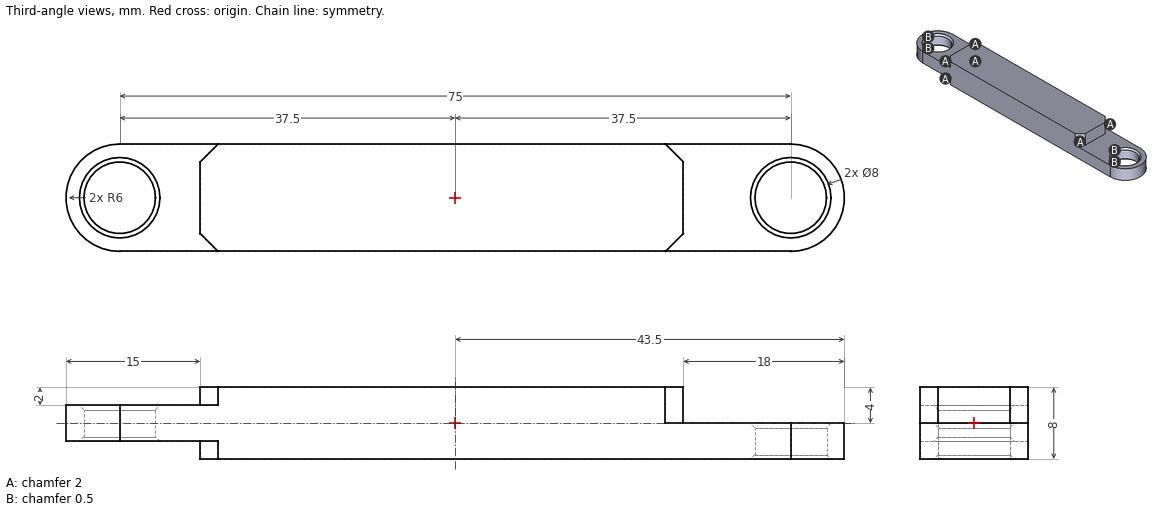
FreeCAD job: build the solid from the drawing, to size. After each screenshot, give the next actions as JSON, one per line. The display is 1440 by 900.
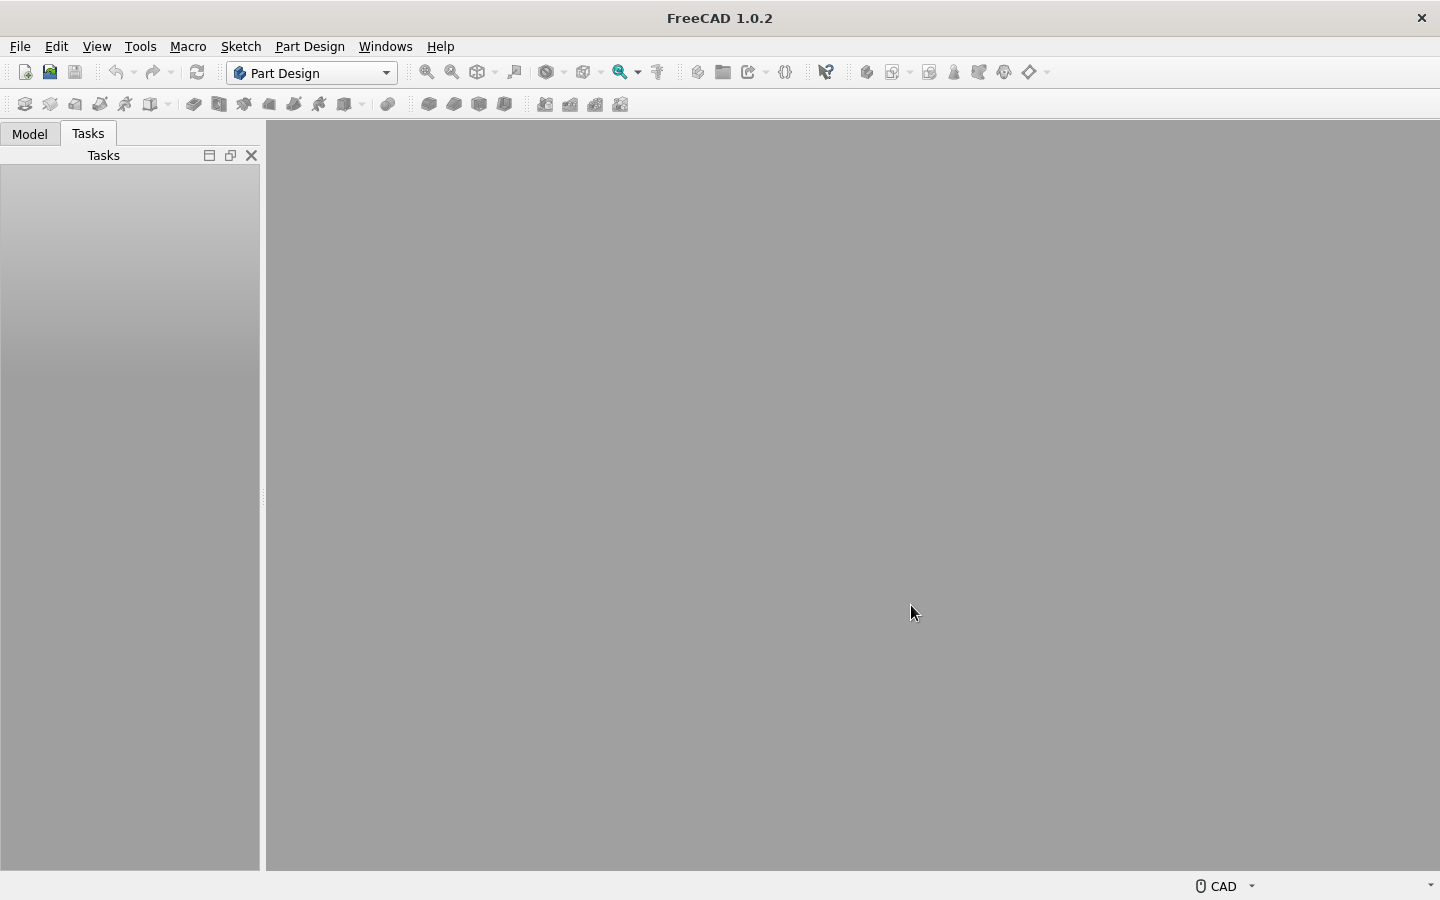
{"action": "left_click", "coordinate": [25, 72]}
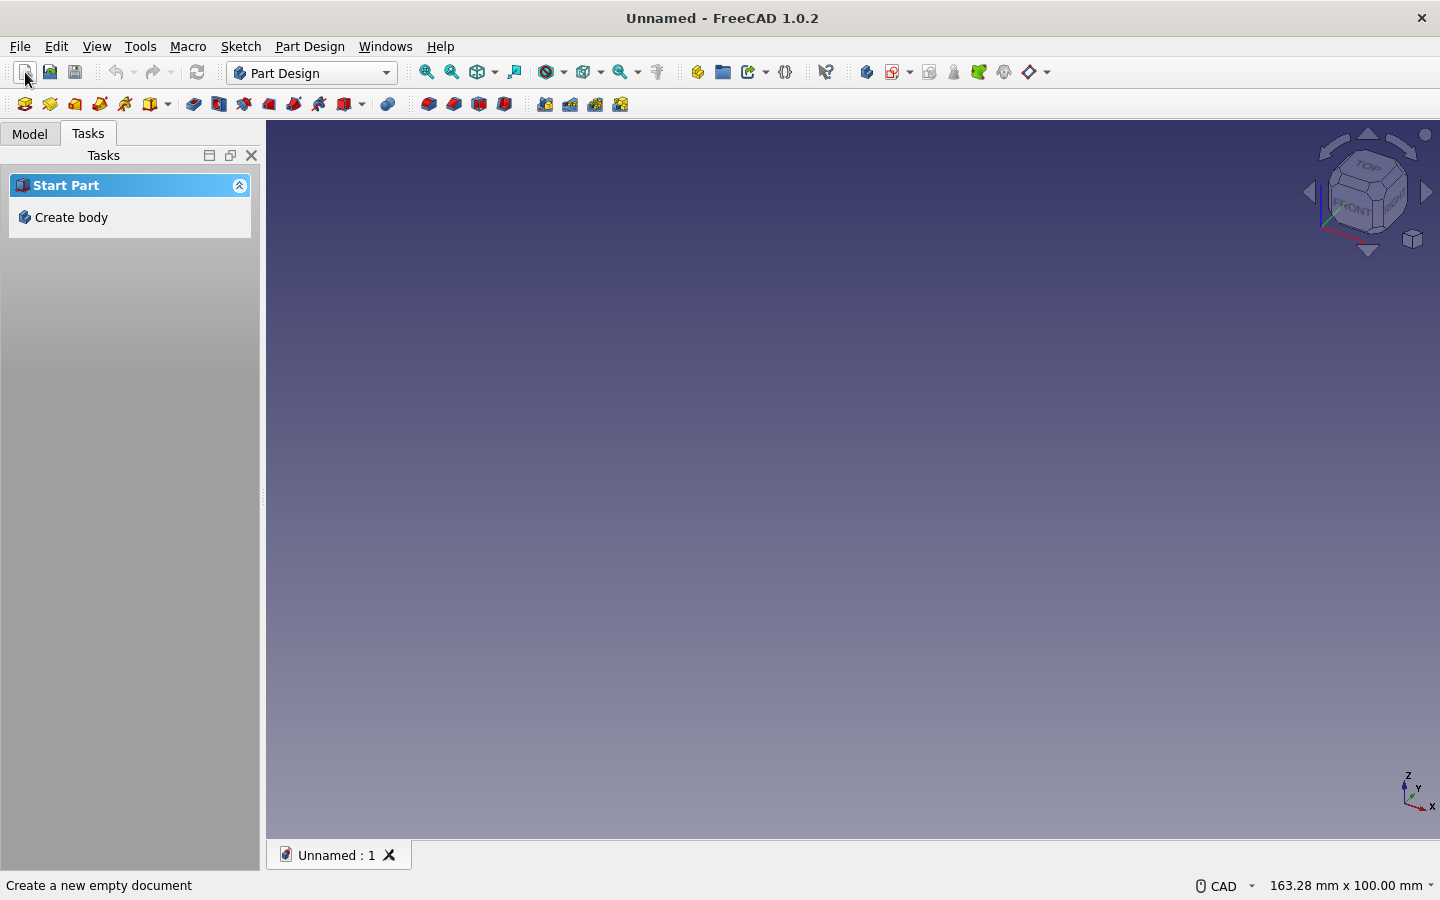
{"action": "left_click", "coordinate": [892, 72]}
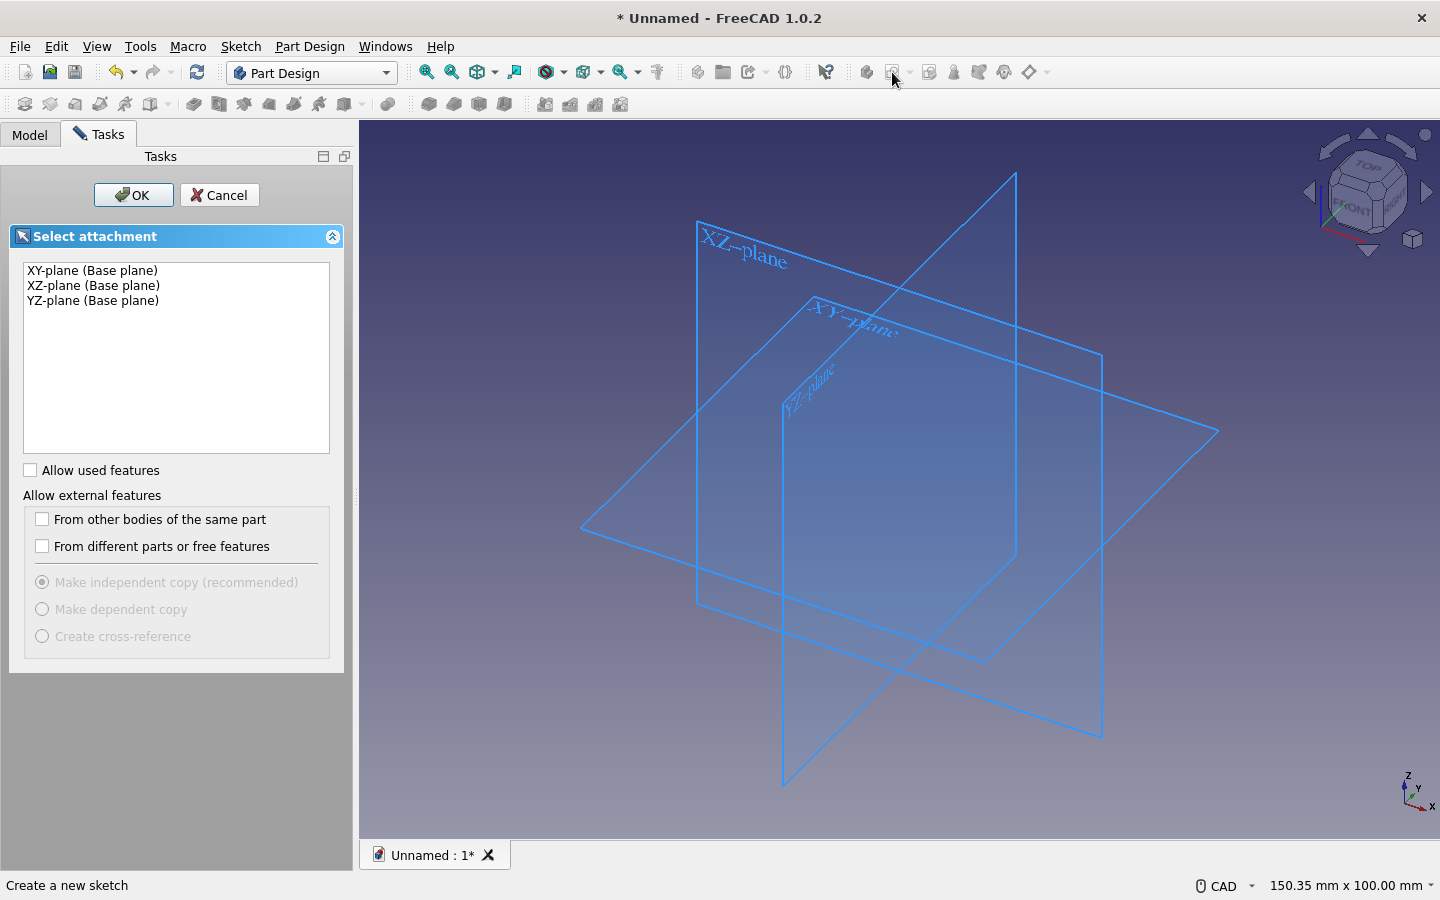
{"action": "left_click", "coordinate": [84, 270]}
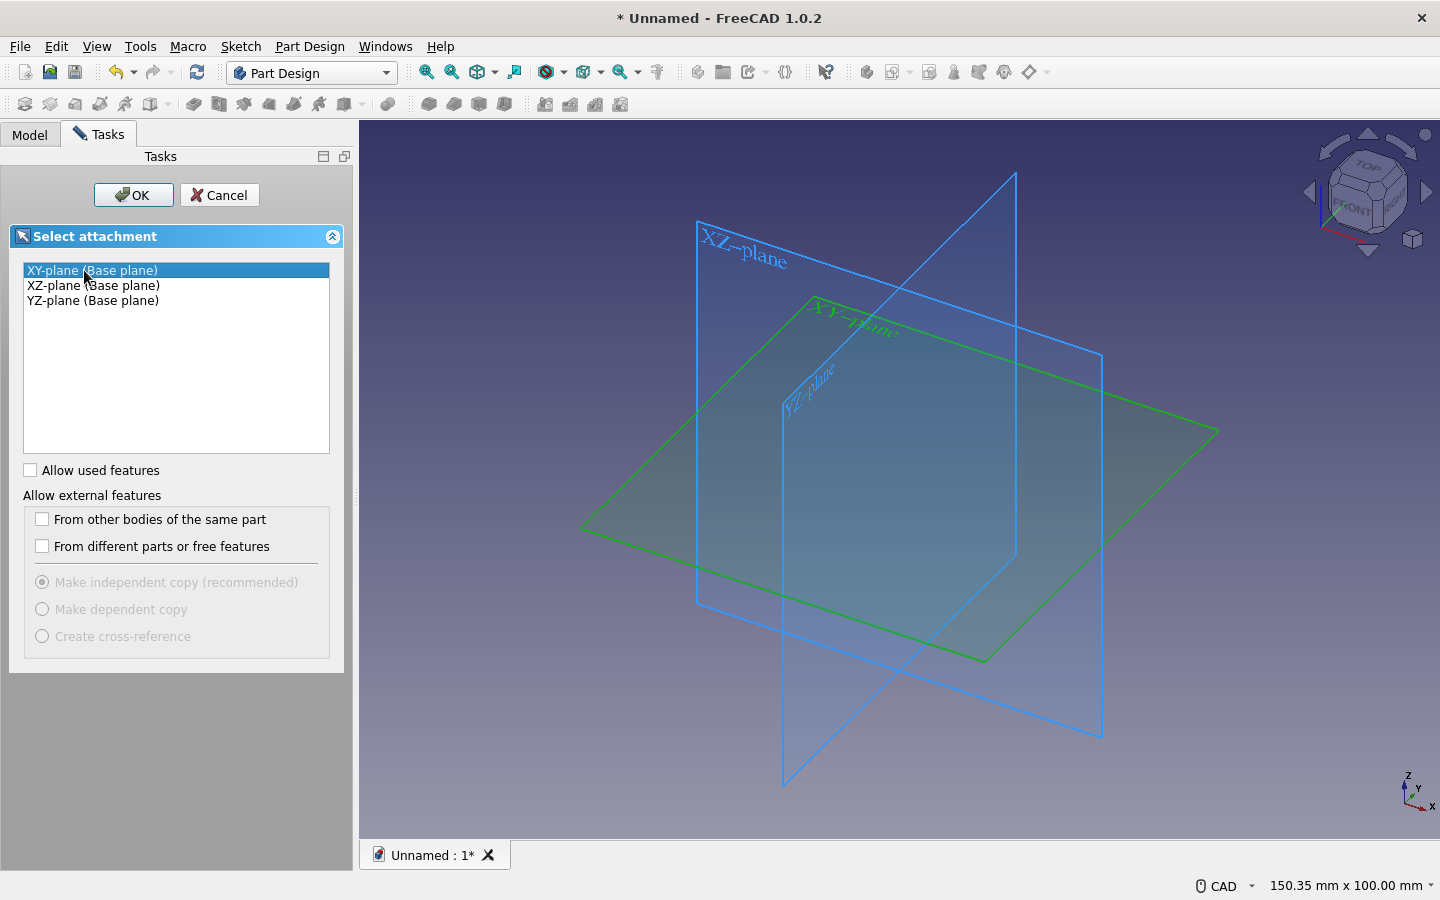
{"action": "left_click", "coordinate": [134, 195]}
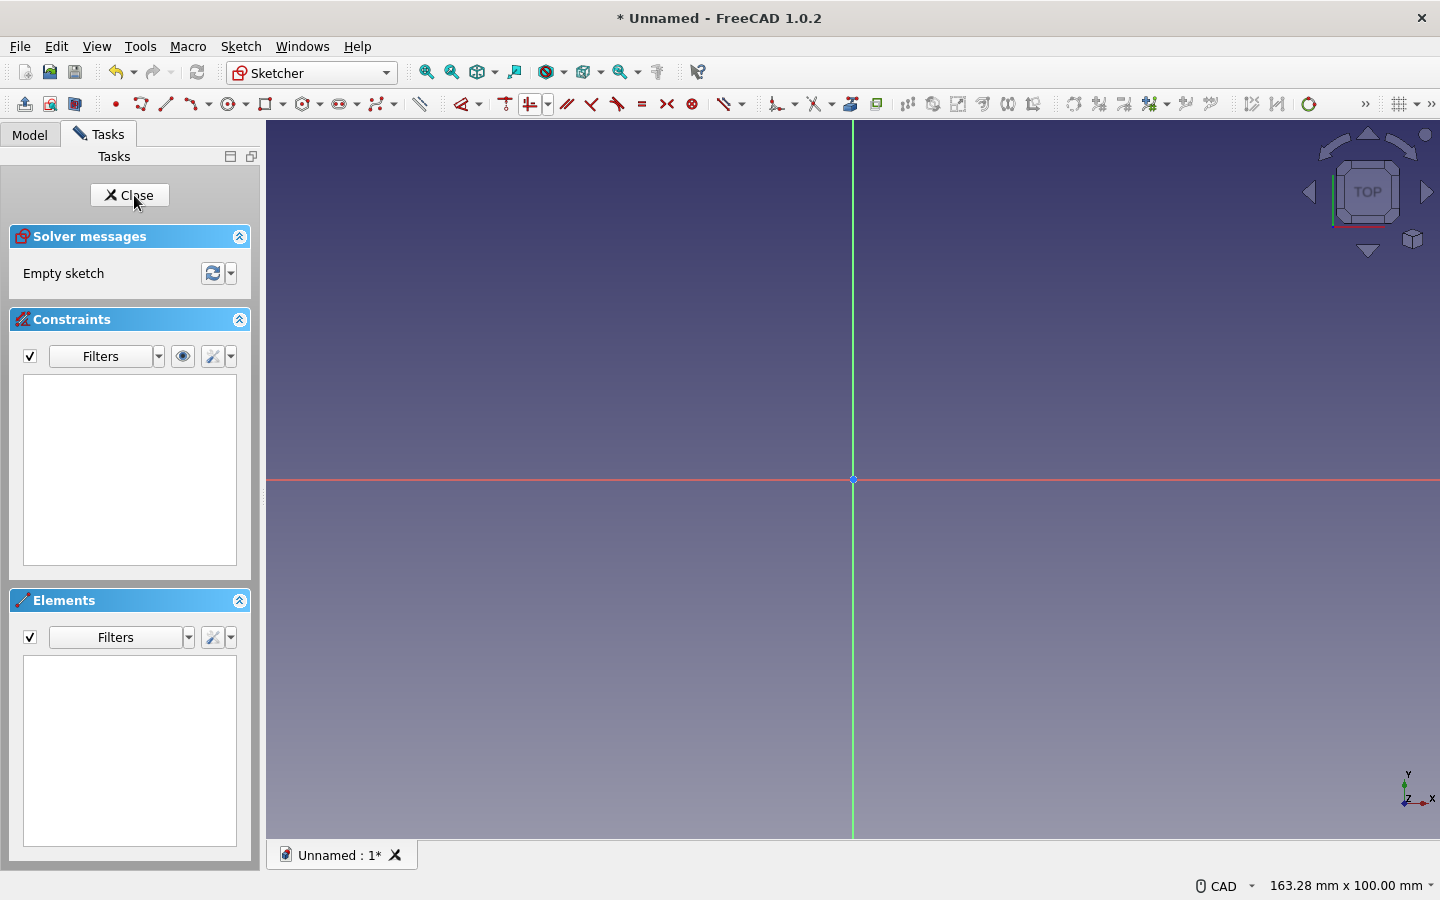
{"action": "key", "text": "g s"}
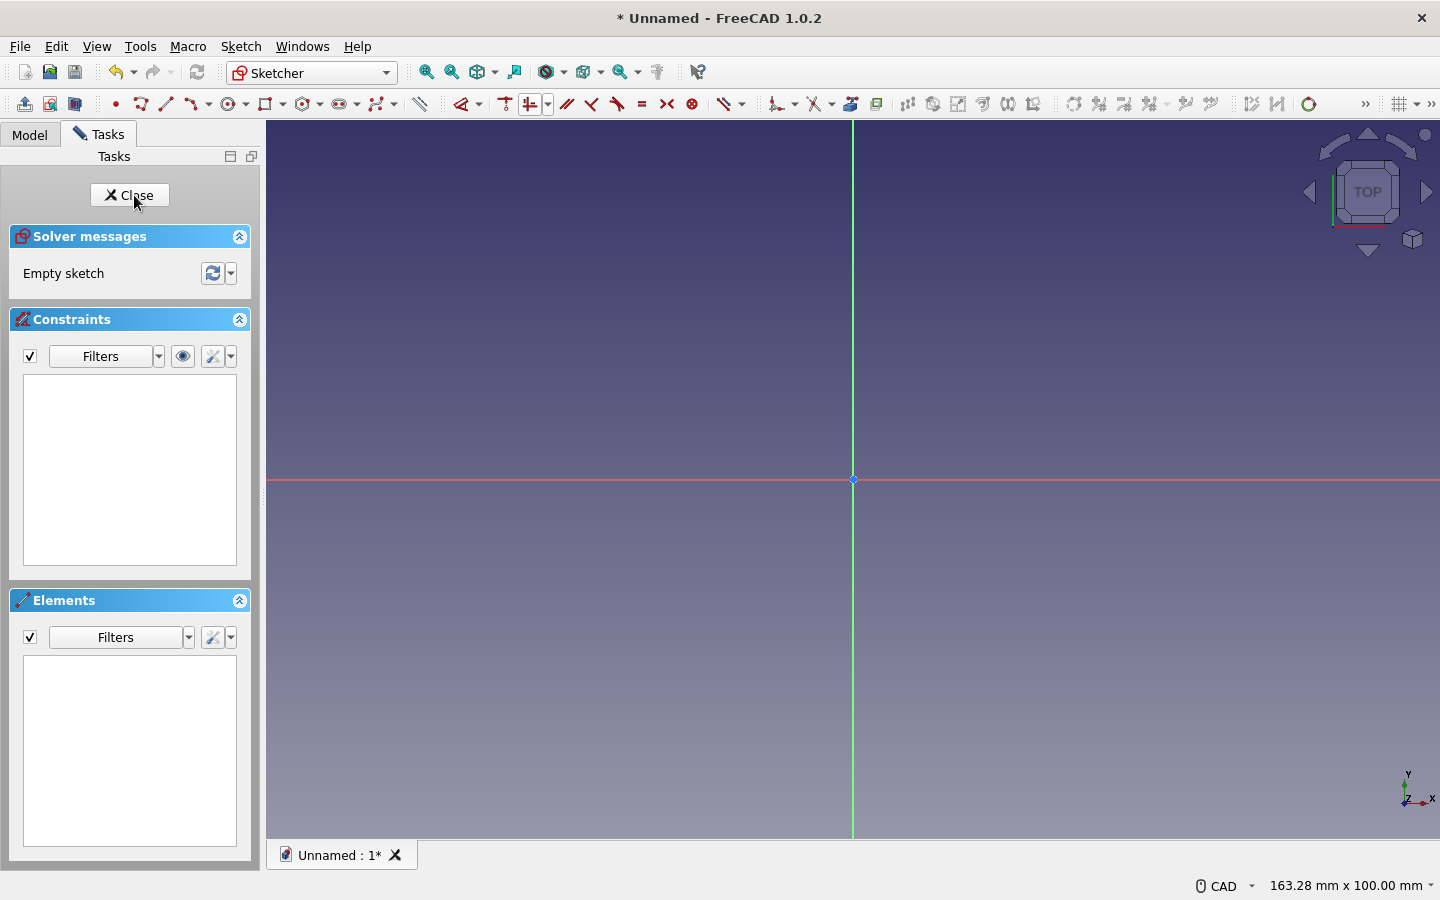
{"action": "left_click", "coordinate": [583, 480]}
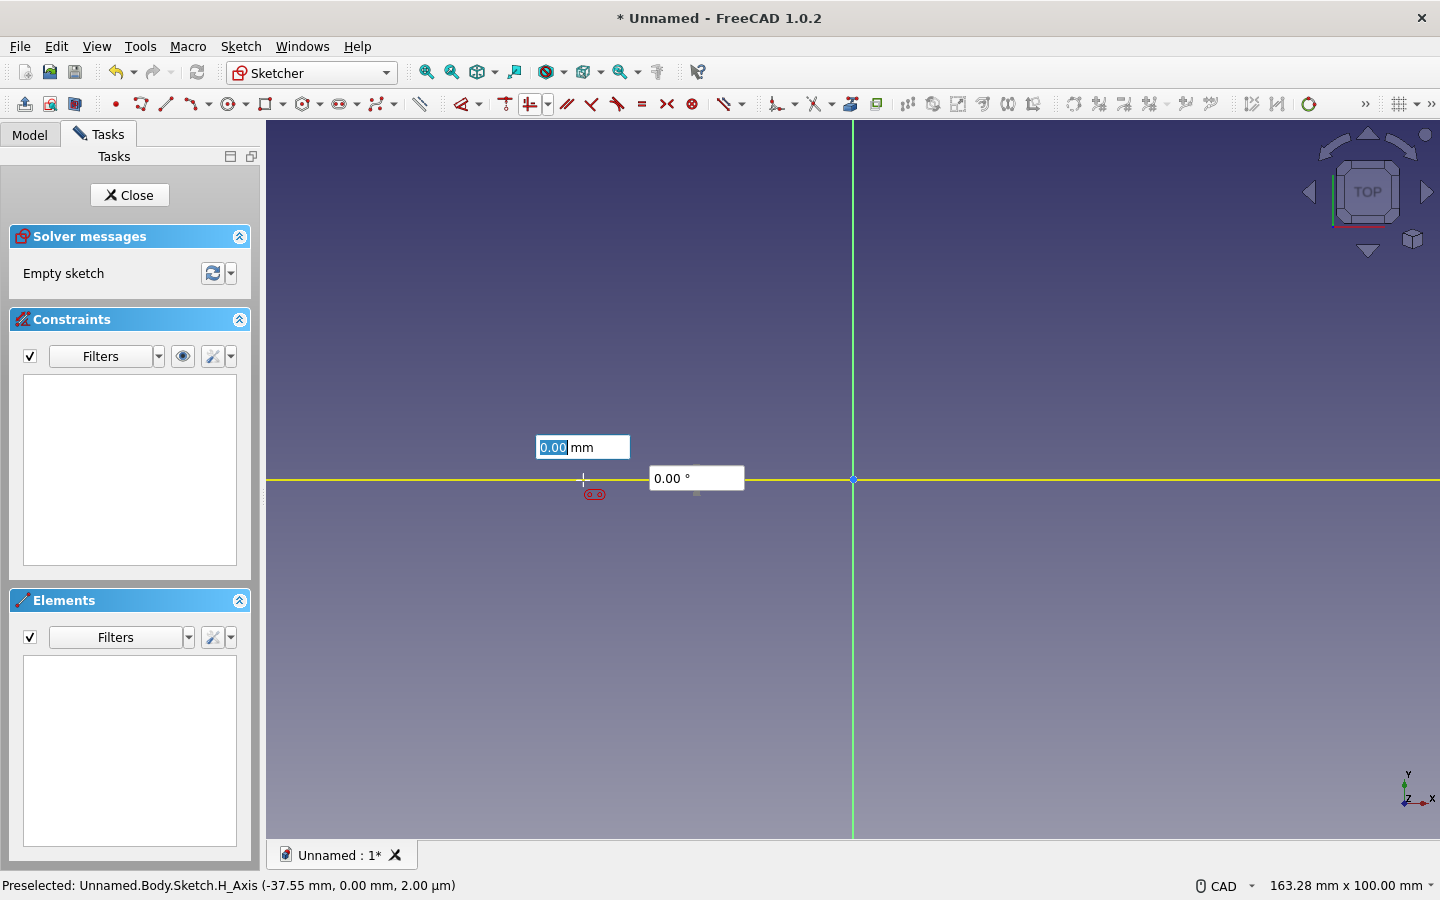
{"action": "left_click", "coordinate": [1123, 470]}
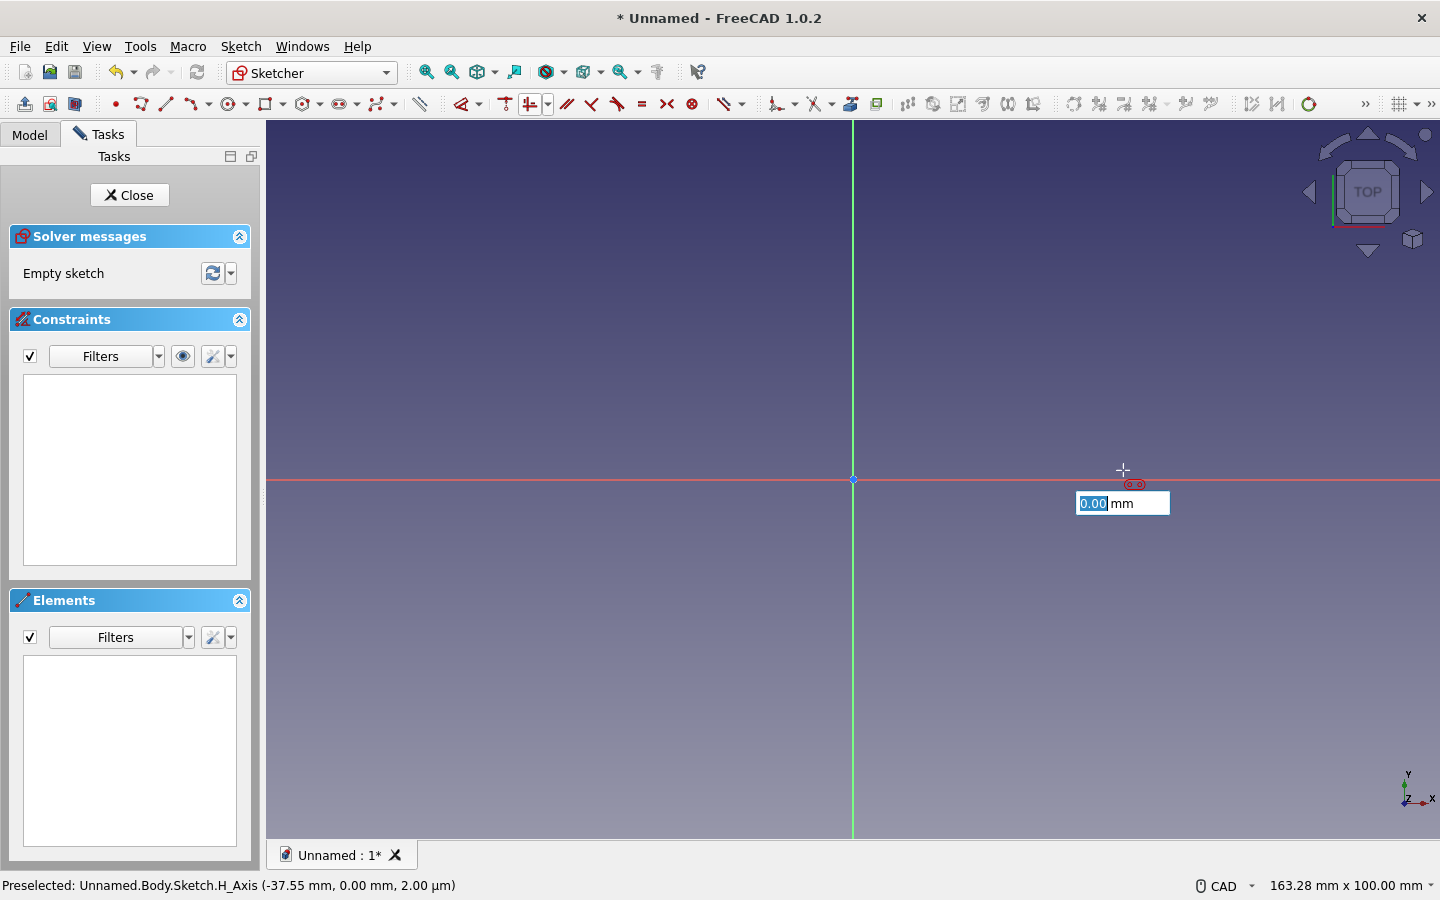
{"action": "left_click", "coordinate": [934, 436]}
{"action": "key", "text": "Escape"}